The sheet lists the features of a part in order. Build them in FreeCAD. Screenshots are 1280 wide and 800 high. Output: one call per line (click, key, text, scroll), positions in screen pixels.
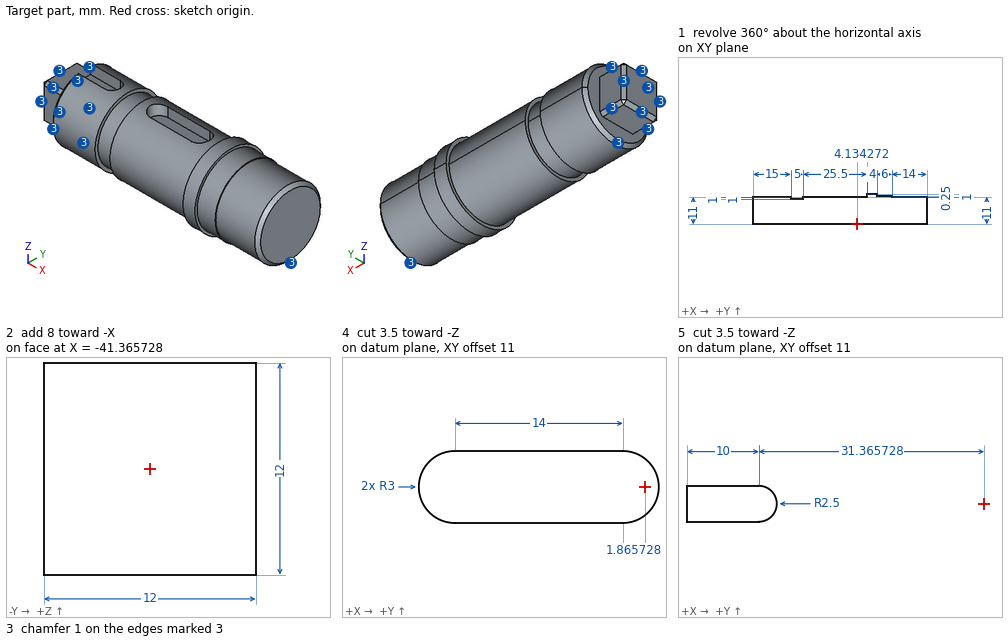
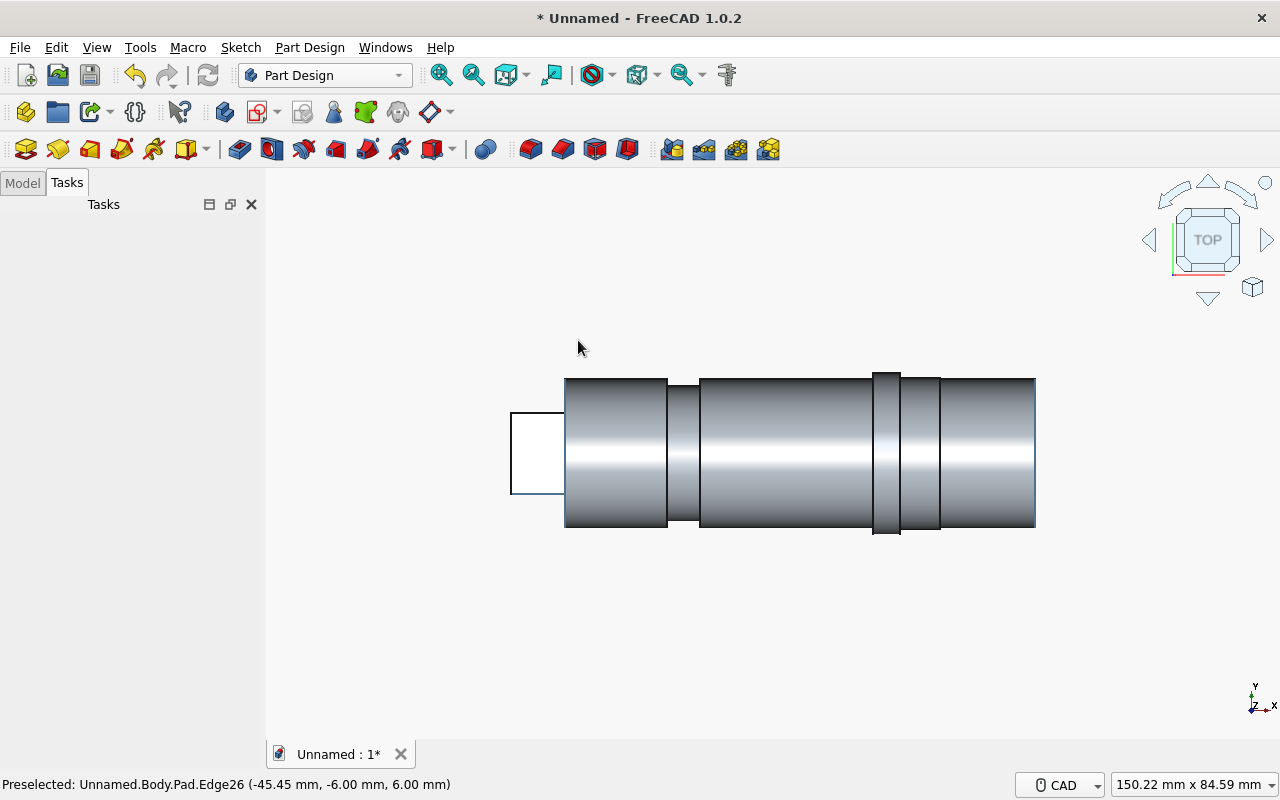
click(538, 412, ctrl)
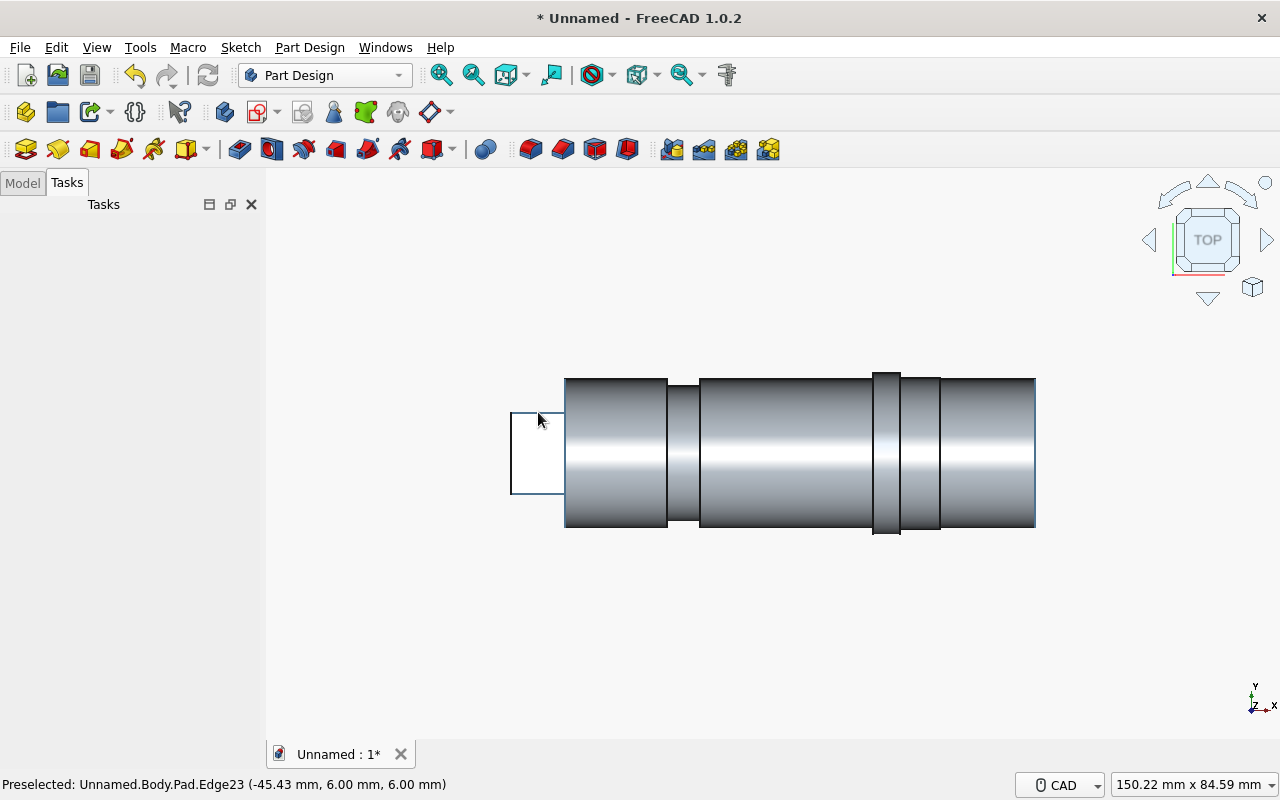
key(1)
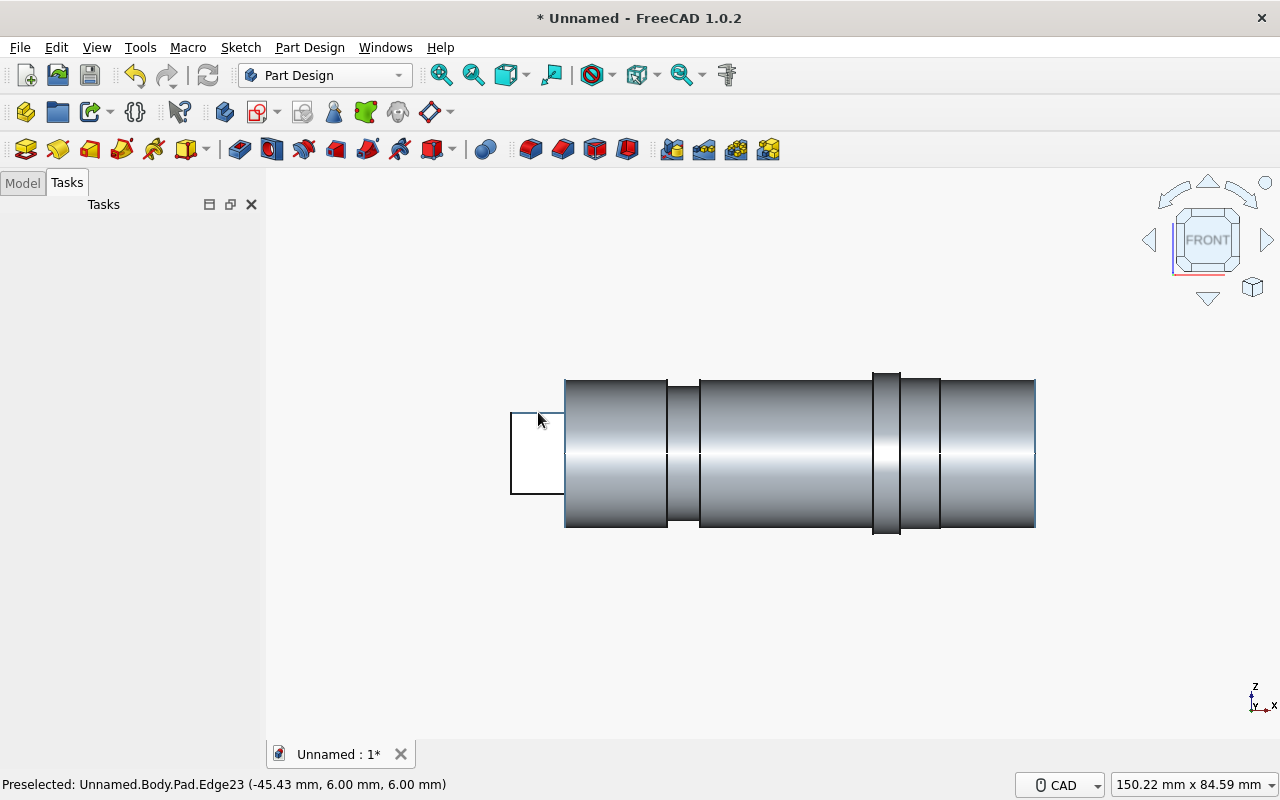
click(538, 493, ctrl)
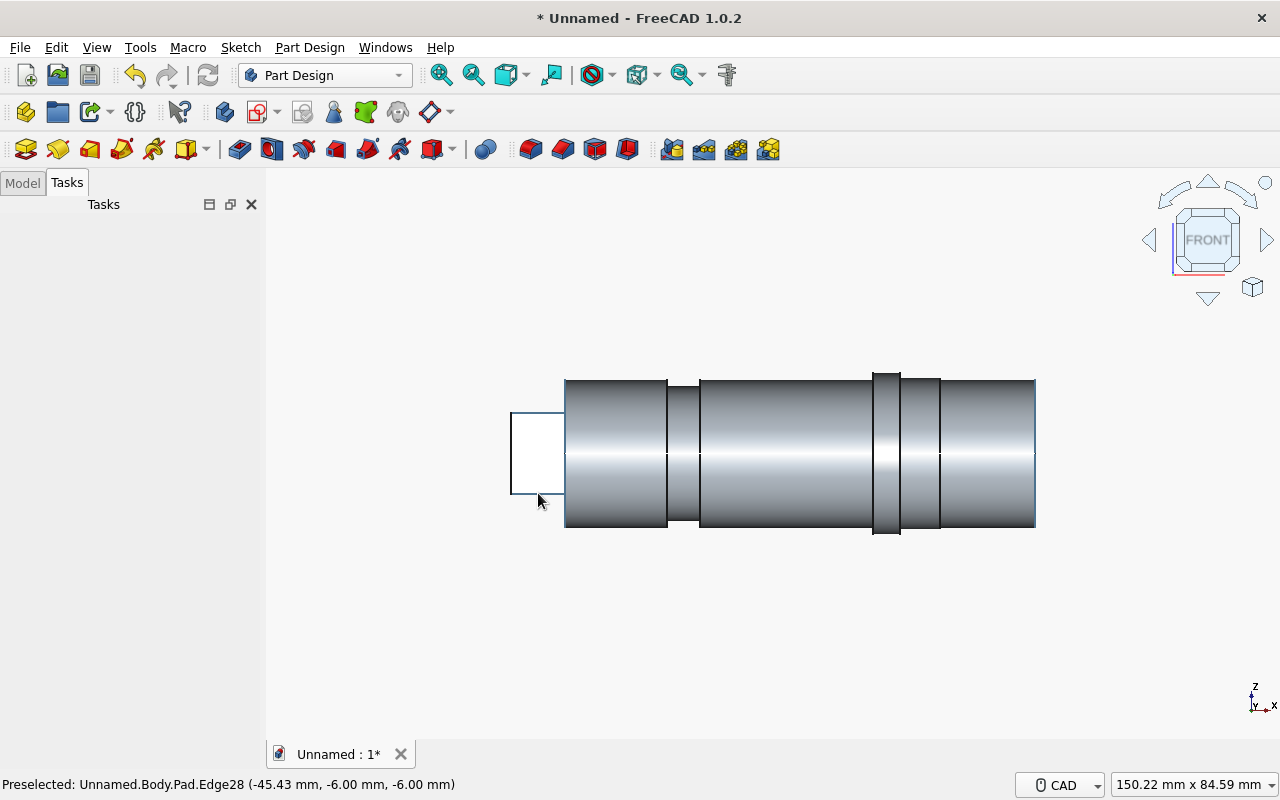
key(3)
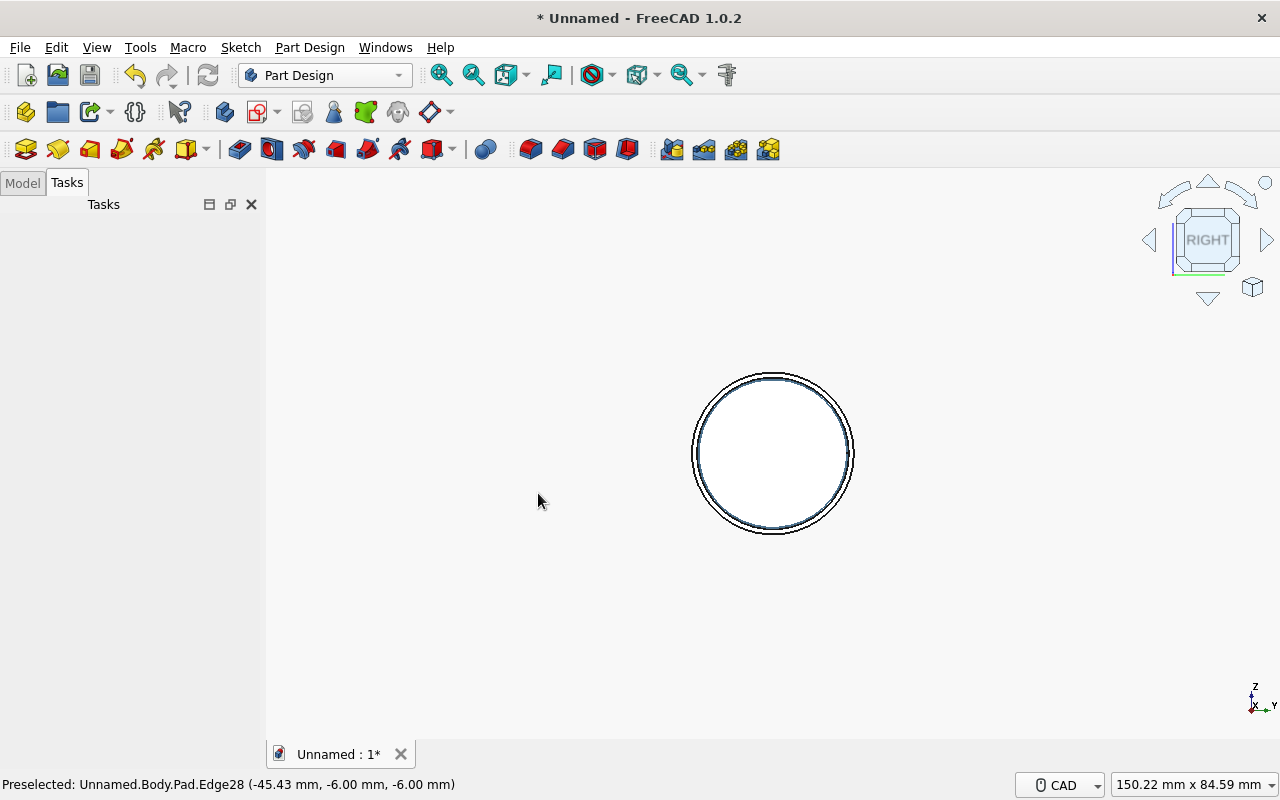
click(442, 76)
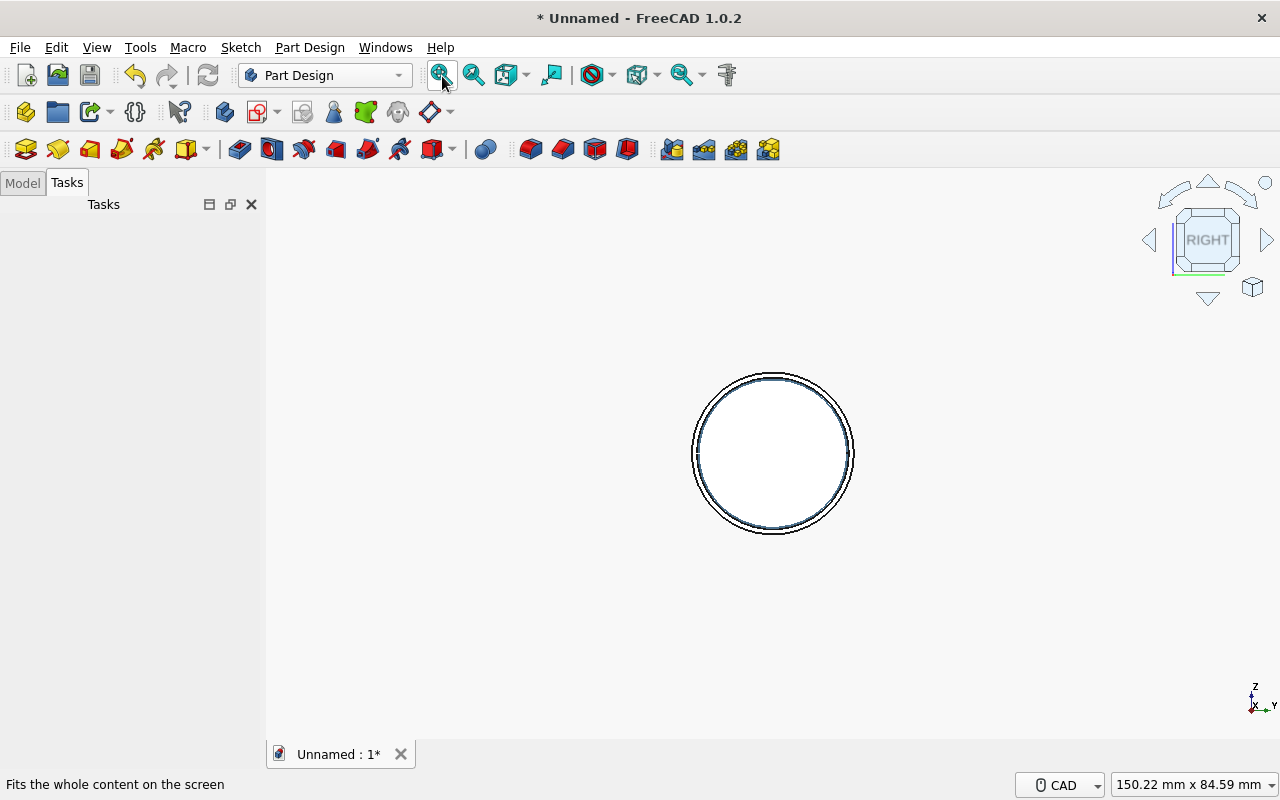
key(5)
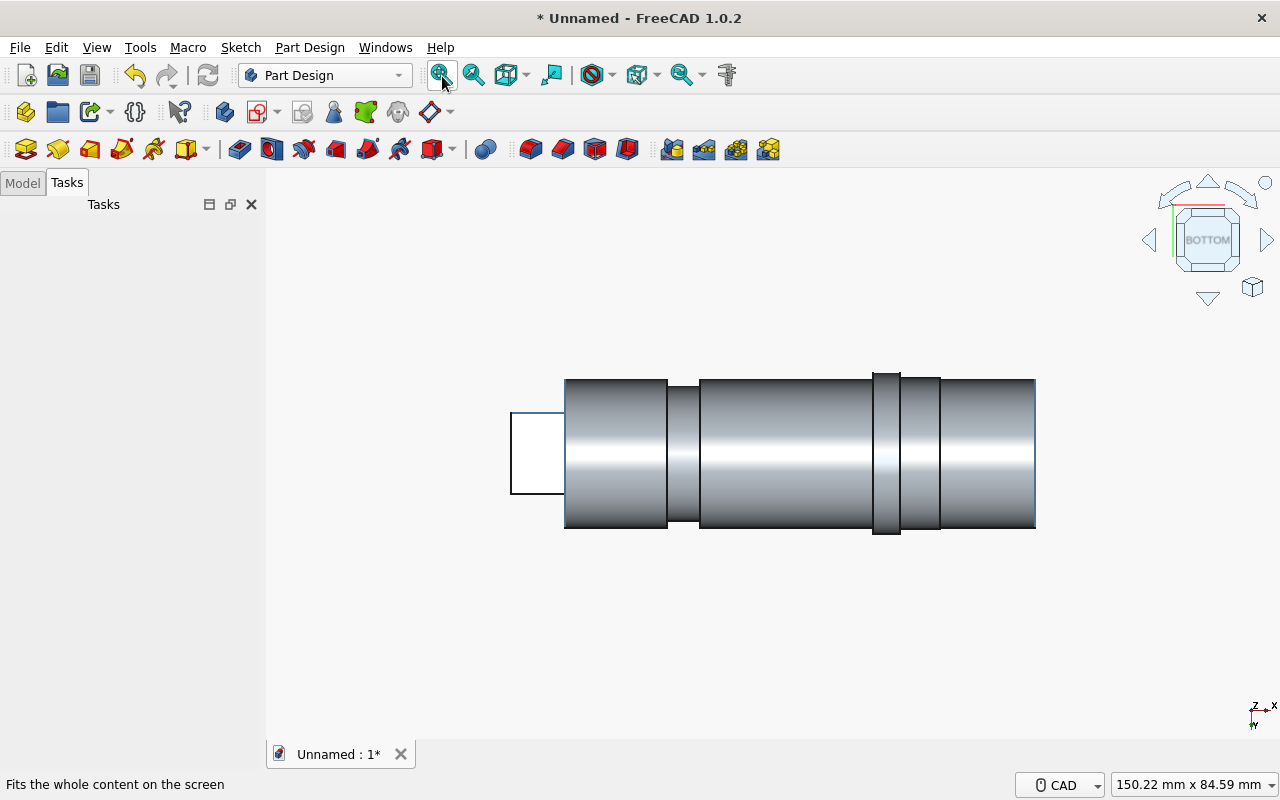
click(538, 493, ctrl)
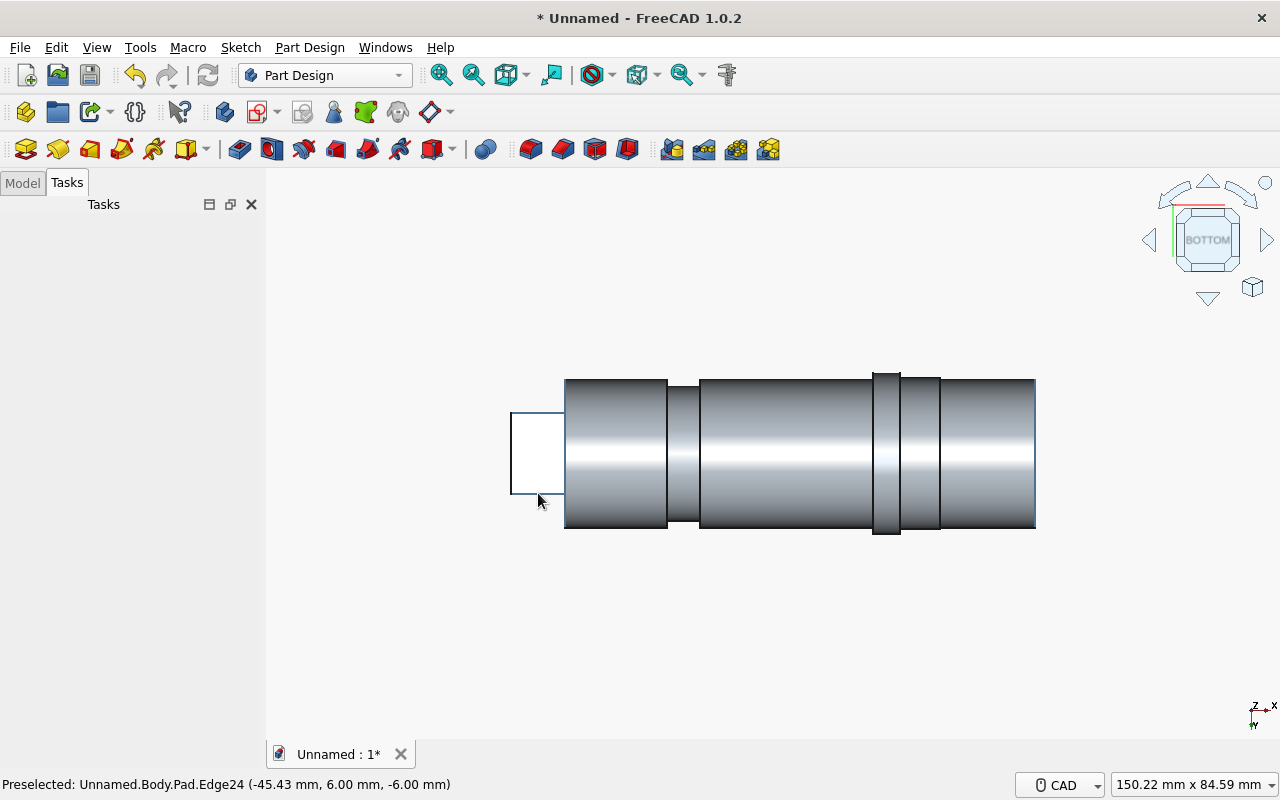
click(564, 150)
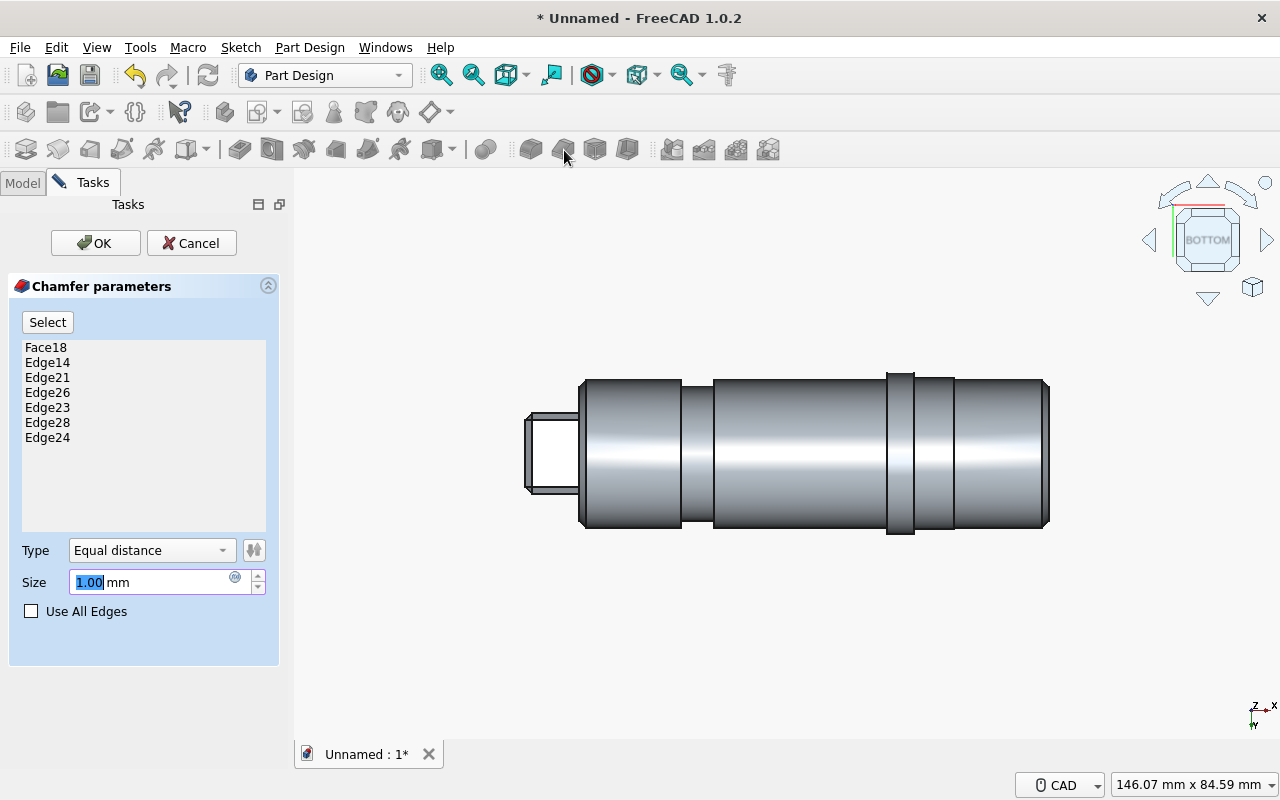
text(1)
key(Tab)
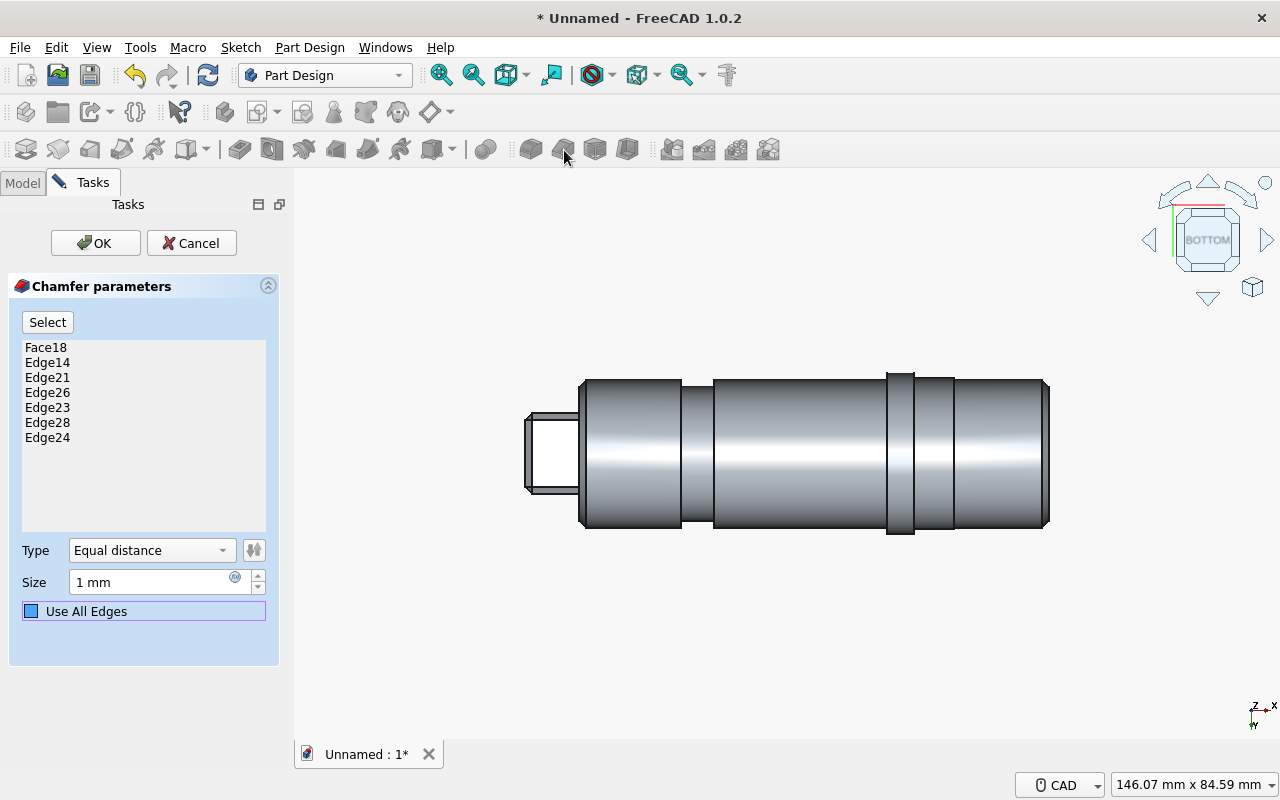
click(96, 243)